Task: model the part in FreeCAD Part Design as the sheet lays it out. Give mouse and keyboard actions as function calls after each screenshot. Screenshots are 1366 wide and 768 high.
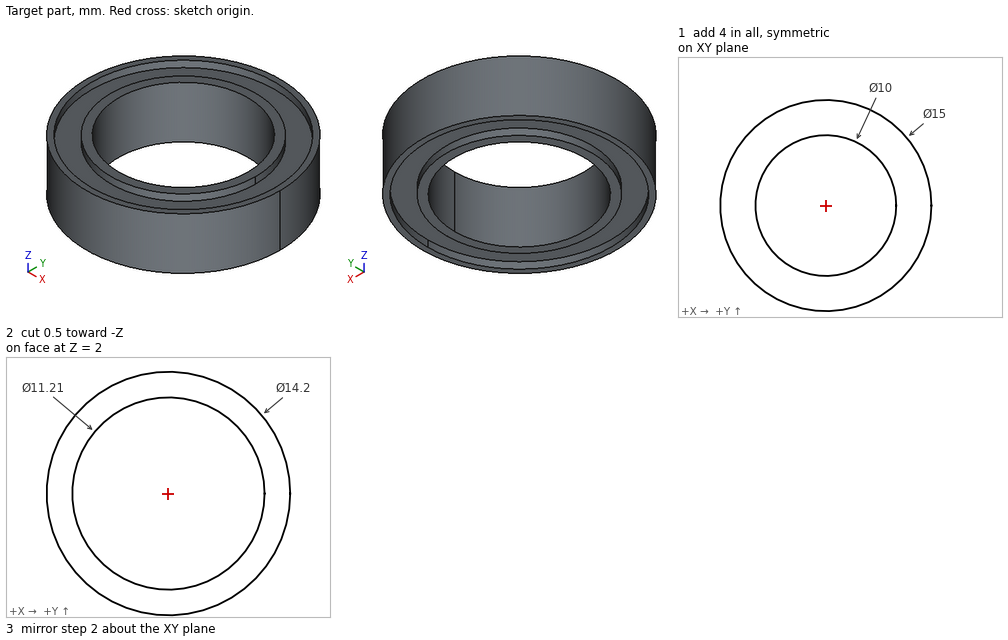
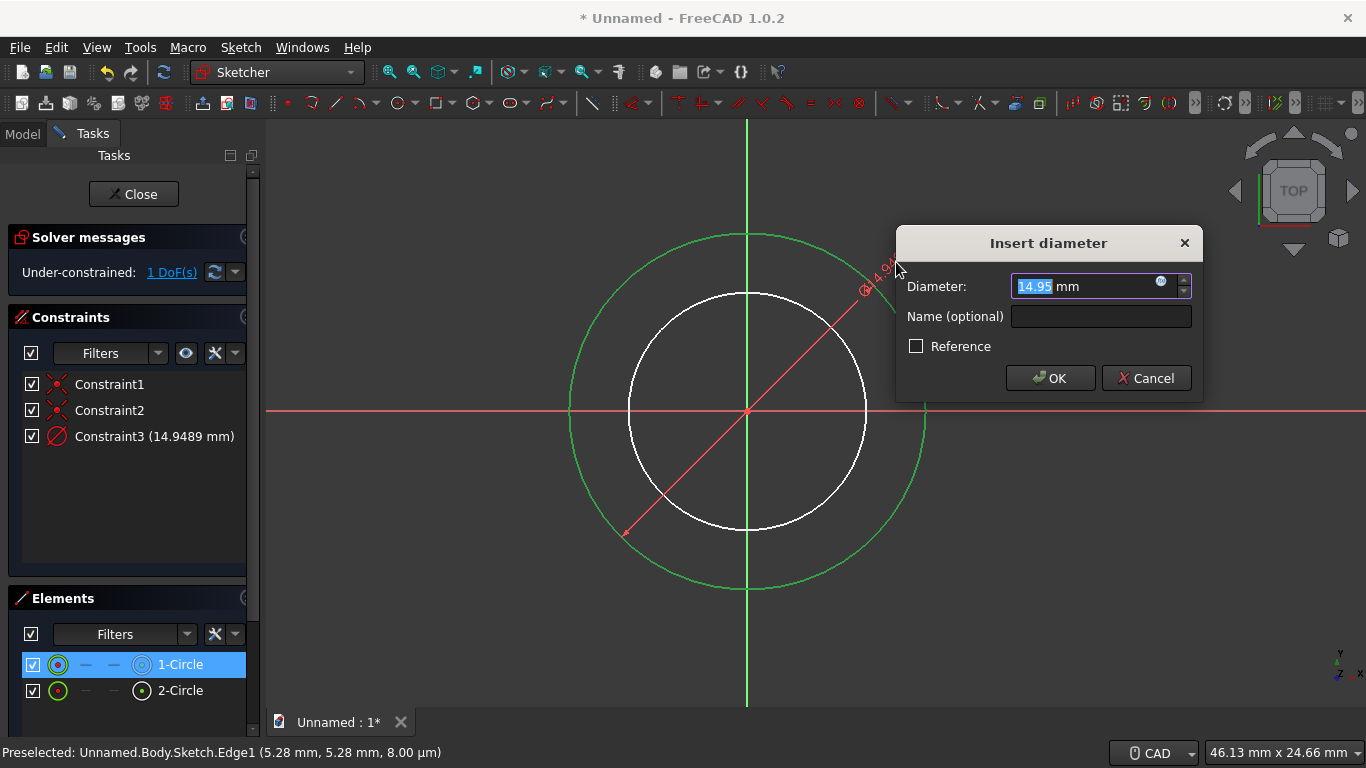
text(15)
key(Return)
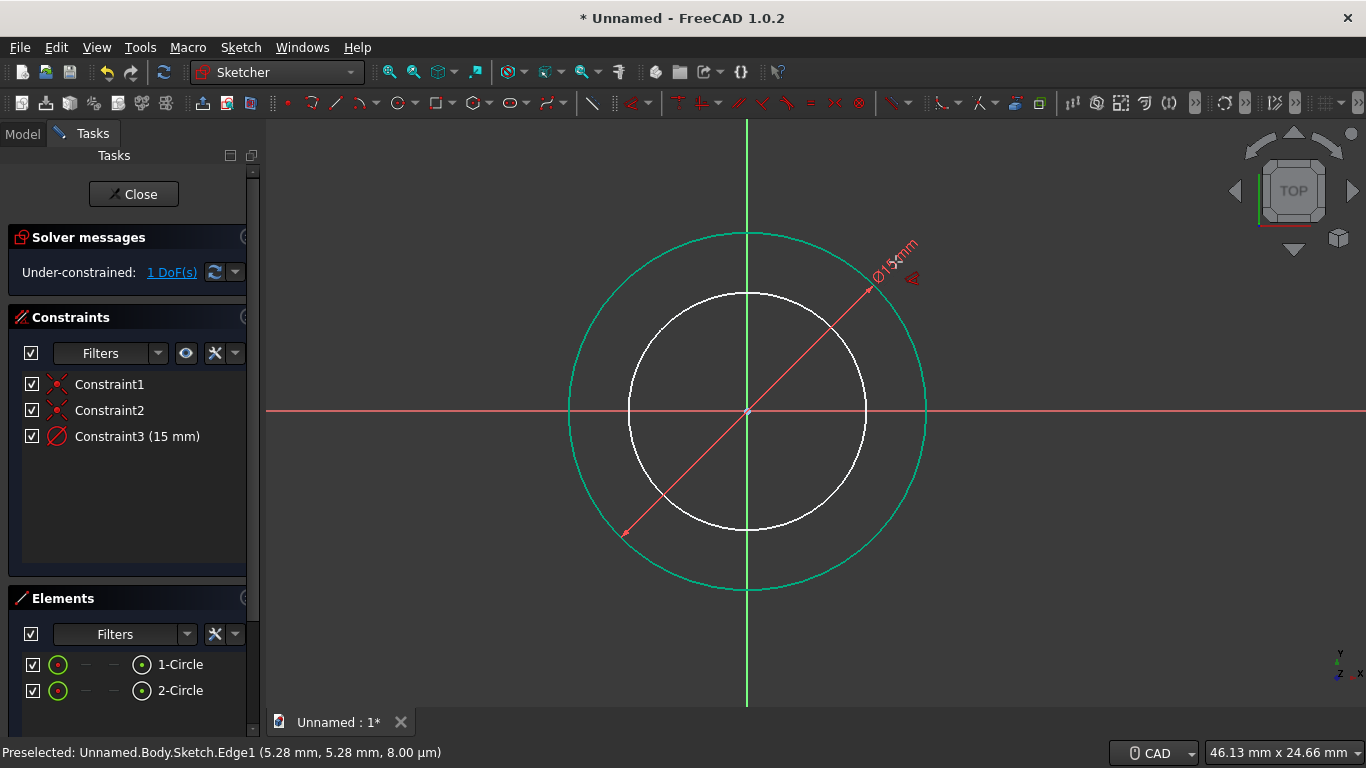
click(831, 327)
click(854, 304)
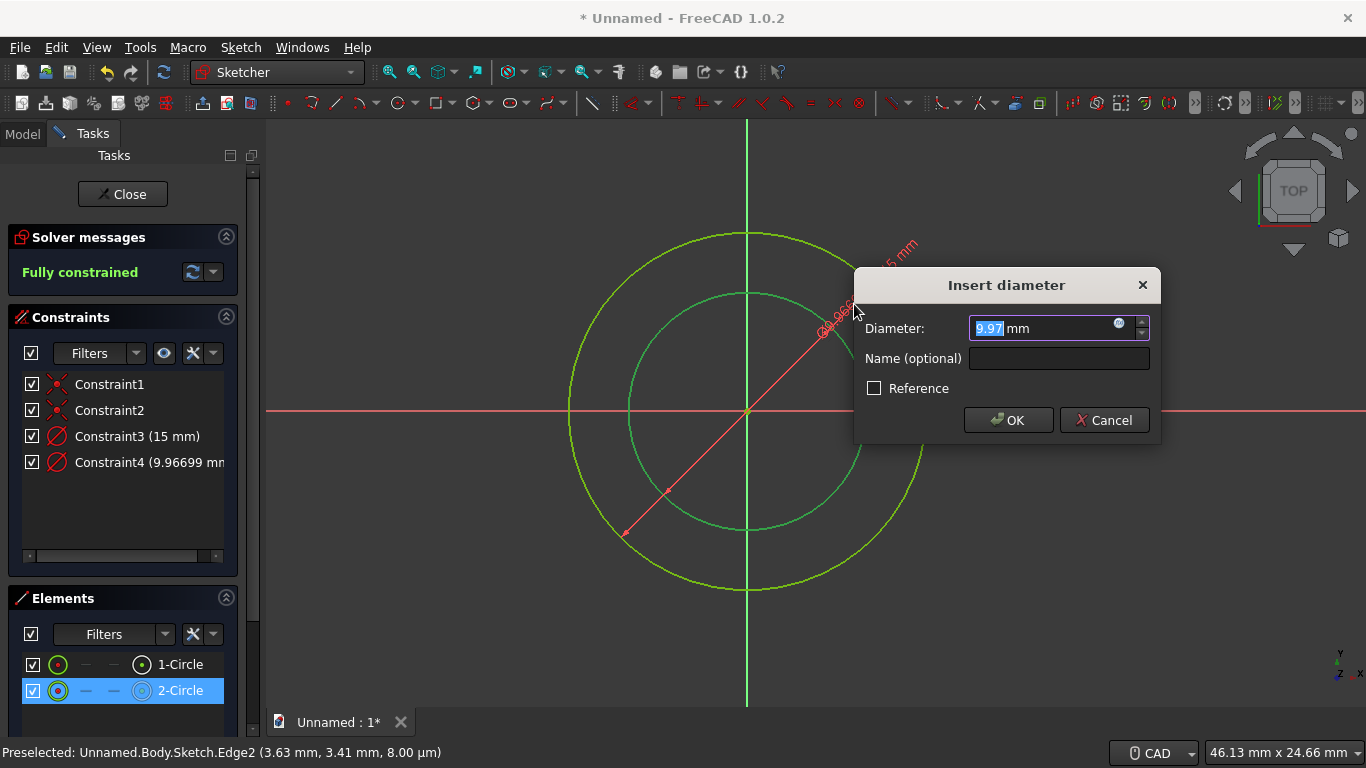
text(10)
key(Return)
key(Escape)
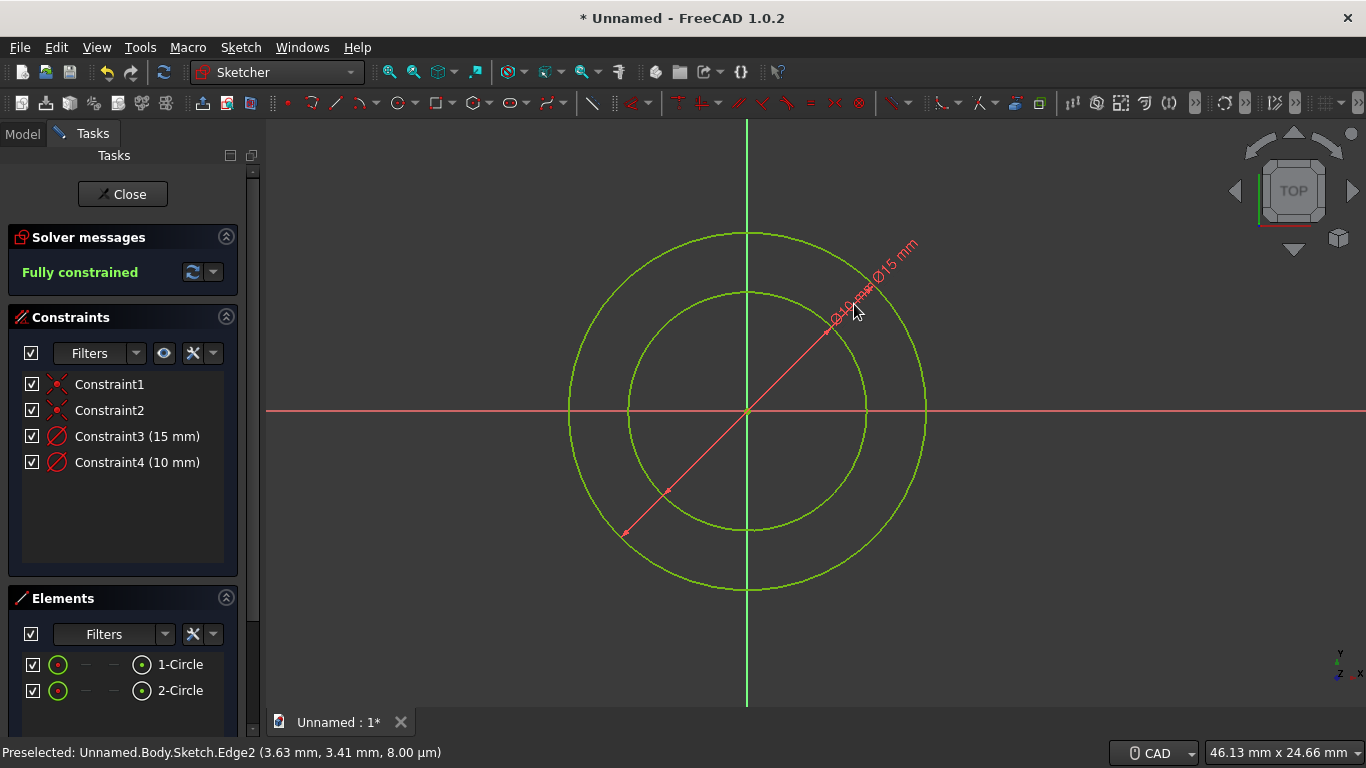
click(123, 194)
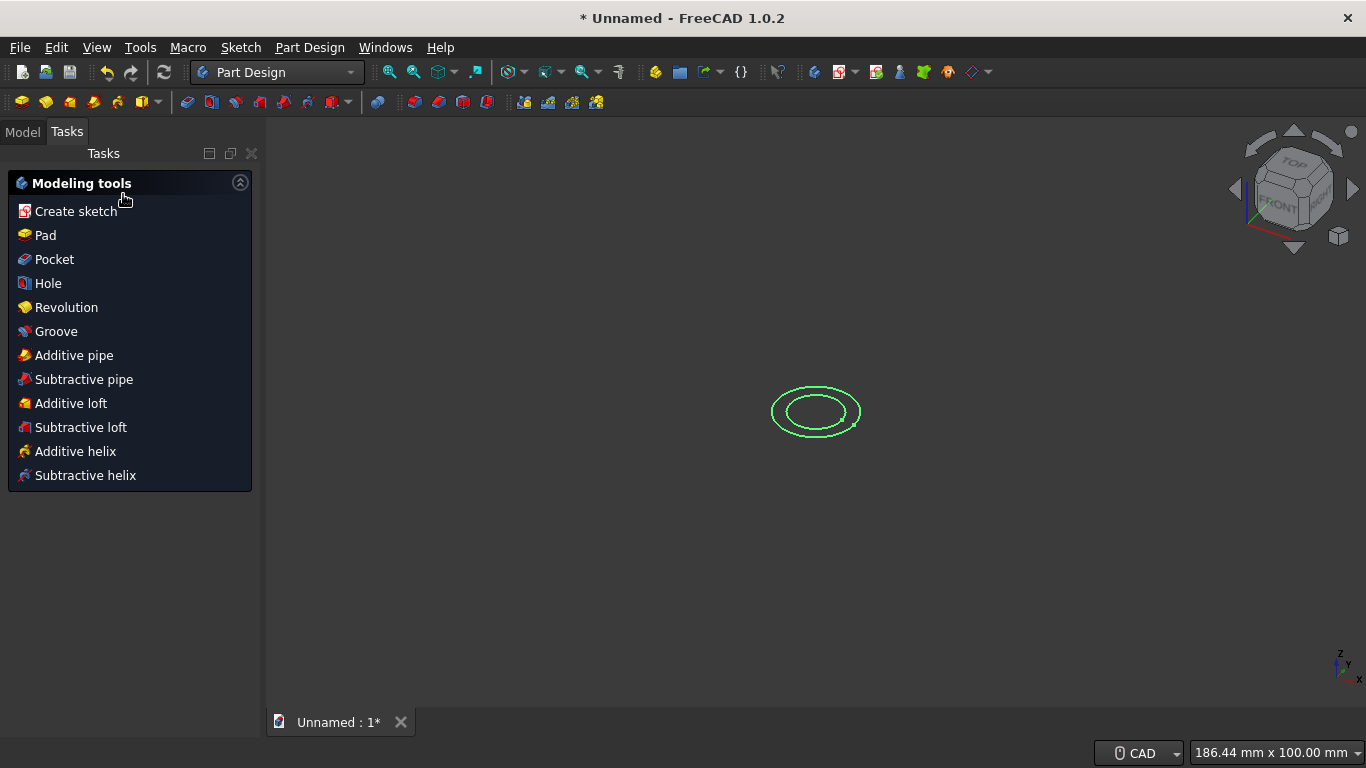
click(22, 102)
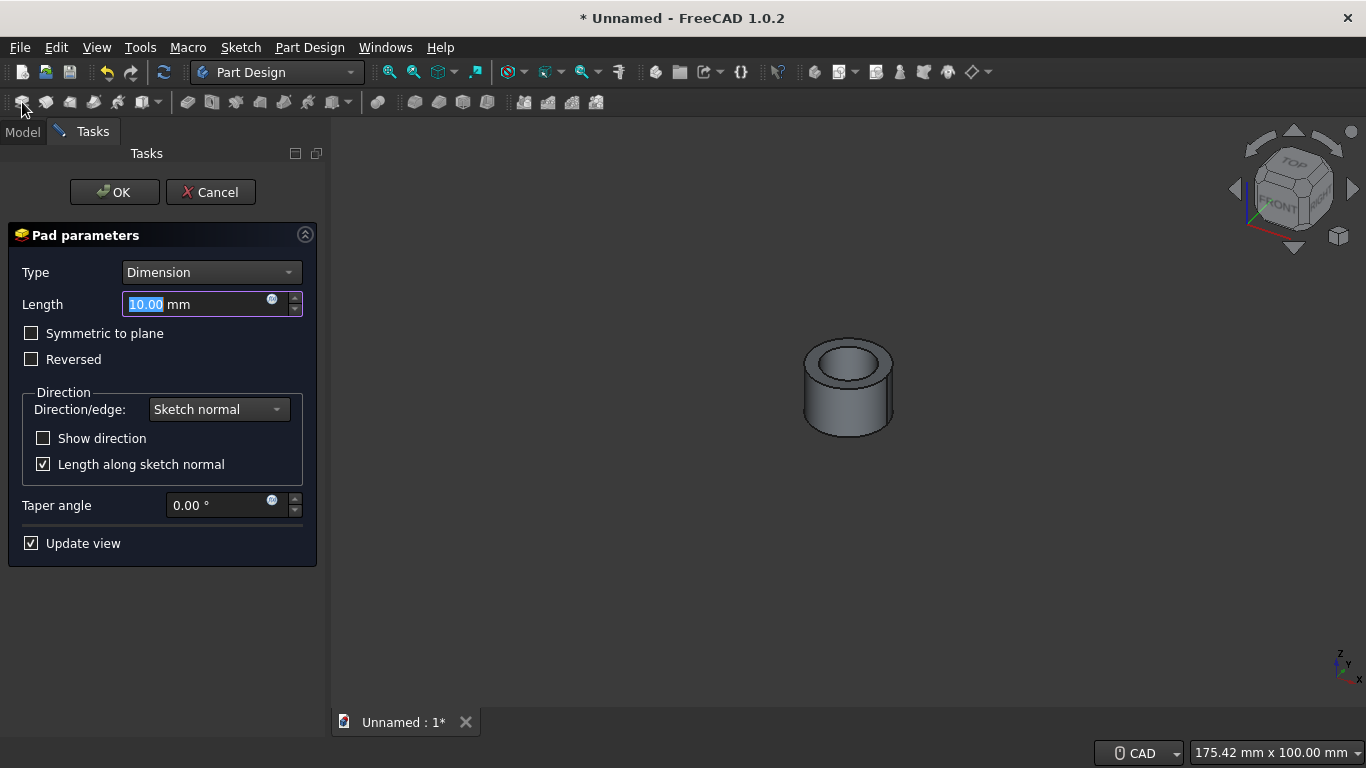
text(4)
key(Tab)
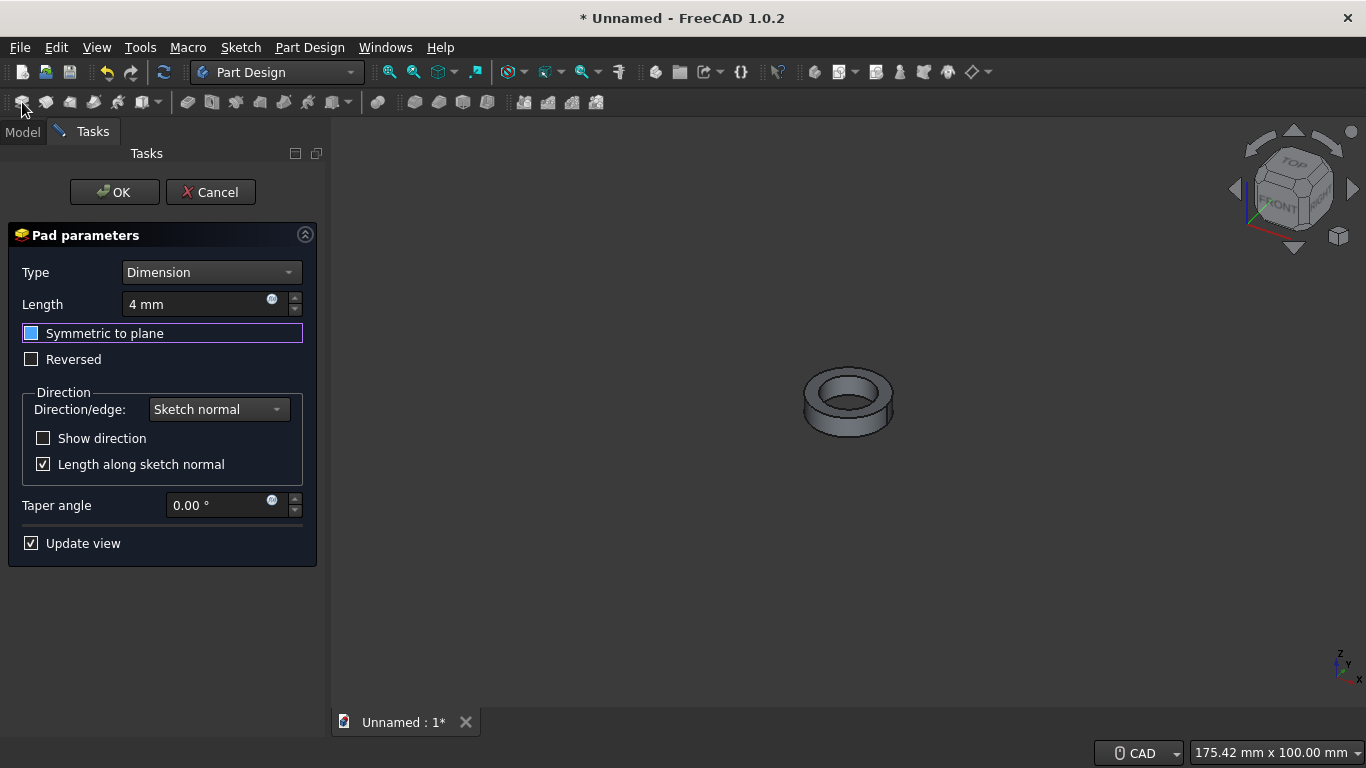
click(30, 333)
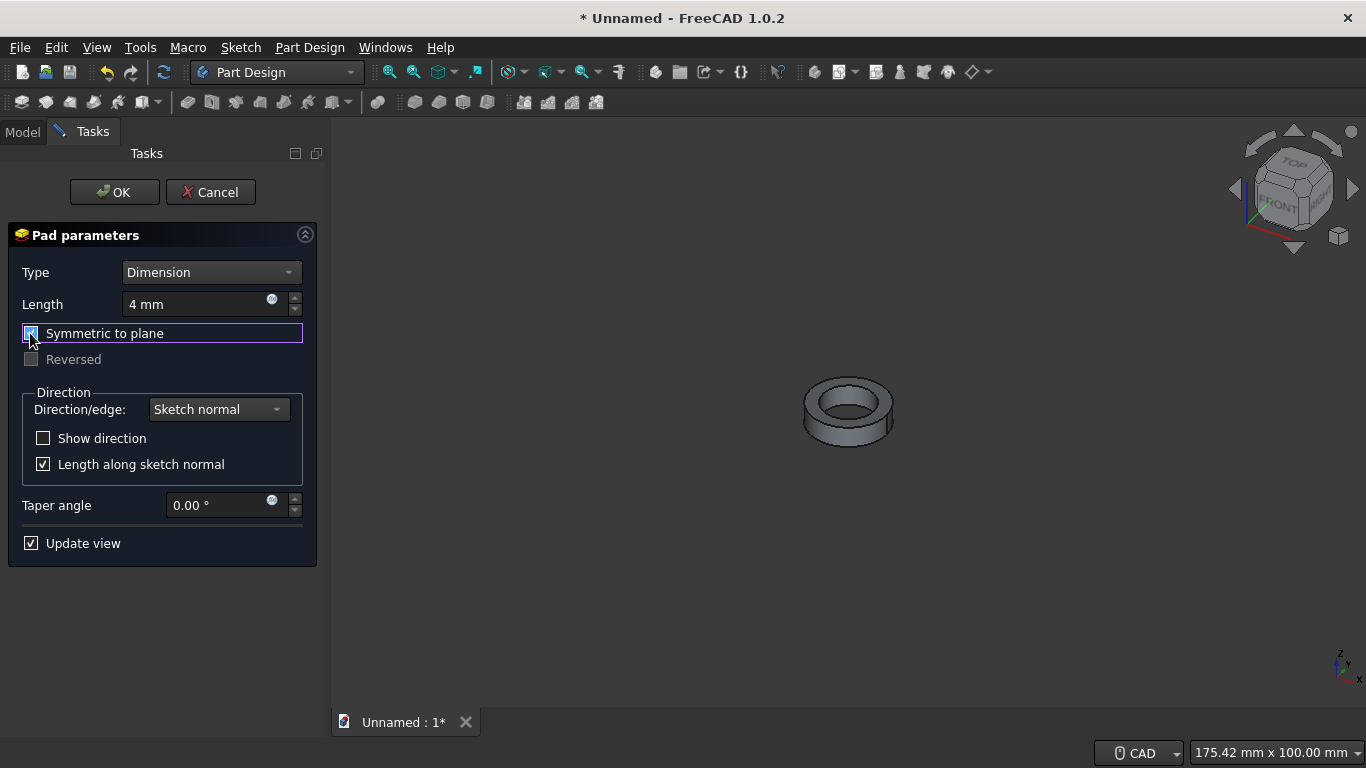
click(115, 192)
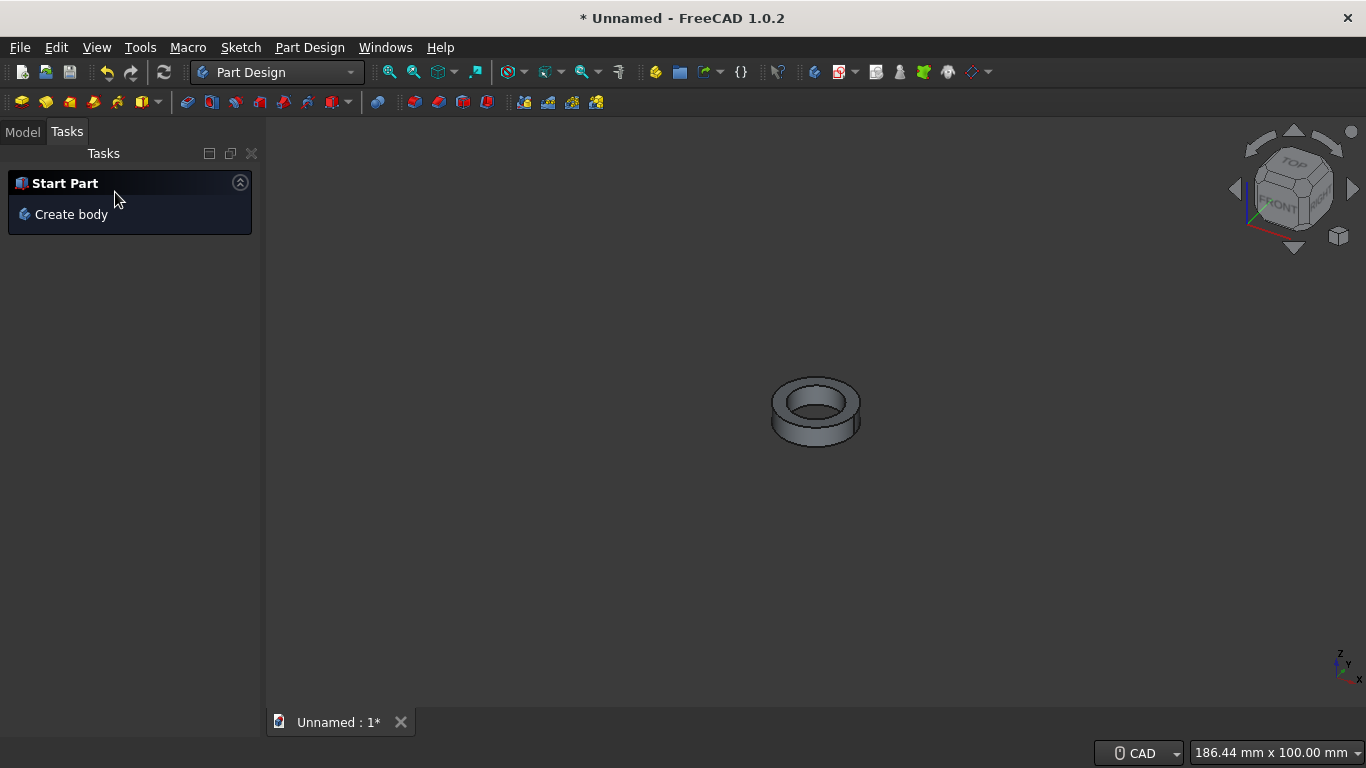
click(390, 72)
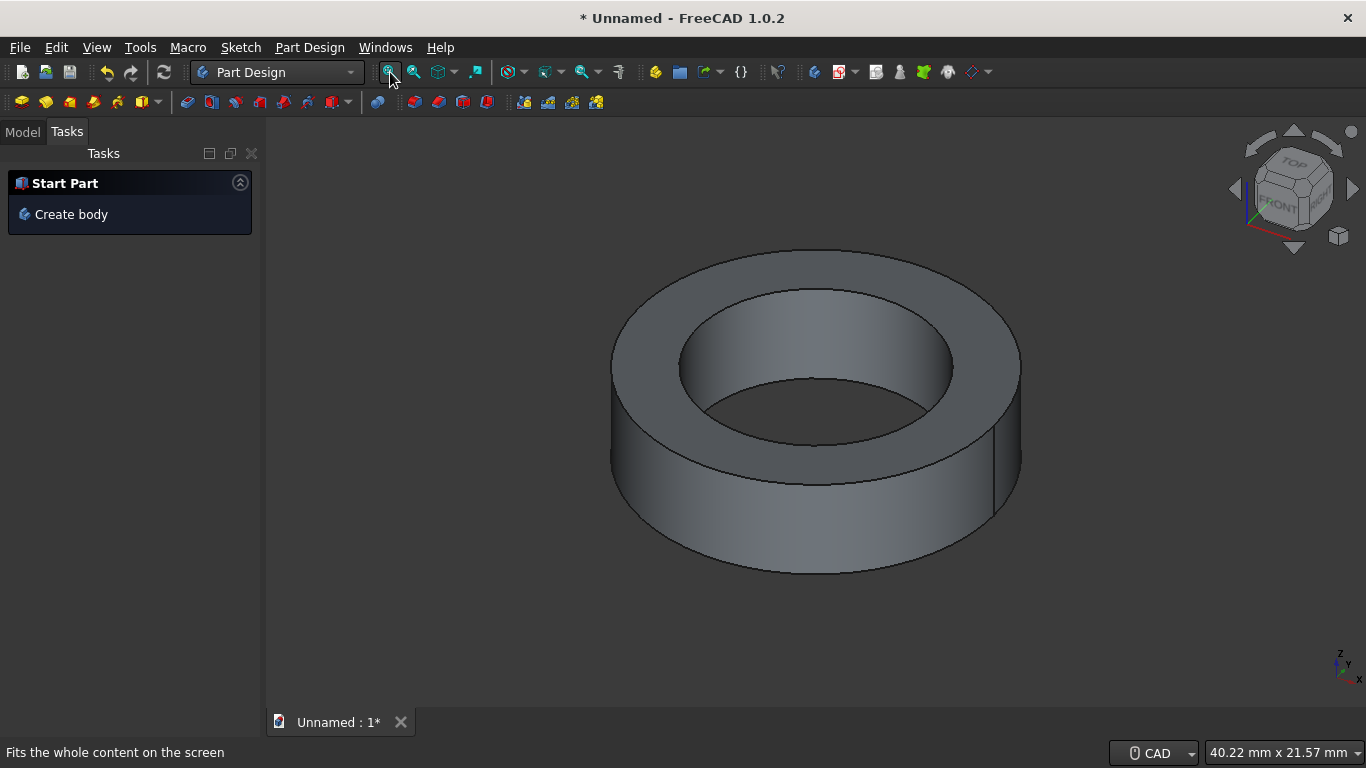
click(968, 417)